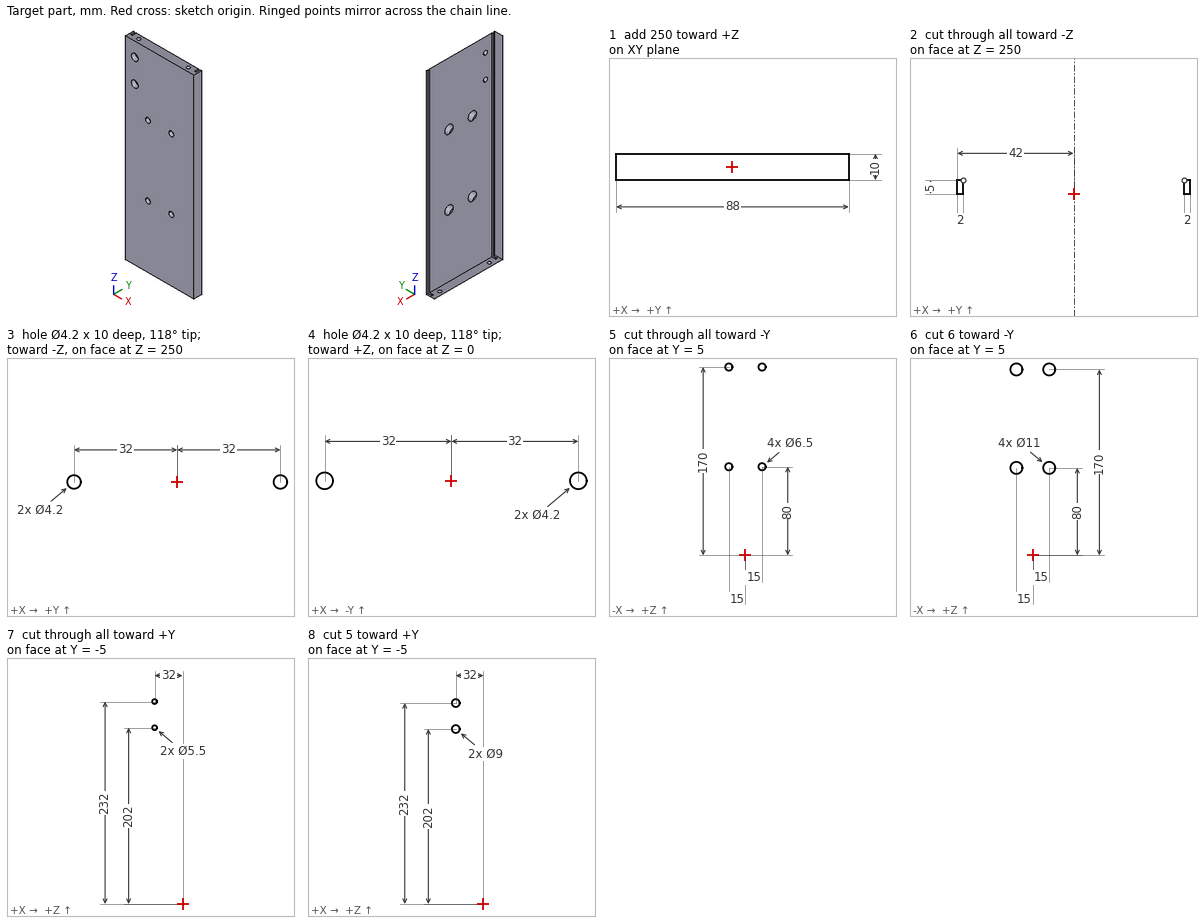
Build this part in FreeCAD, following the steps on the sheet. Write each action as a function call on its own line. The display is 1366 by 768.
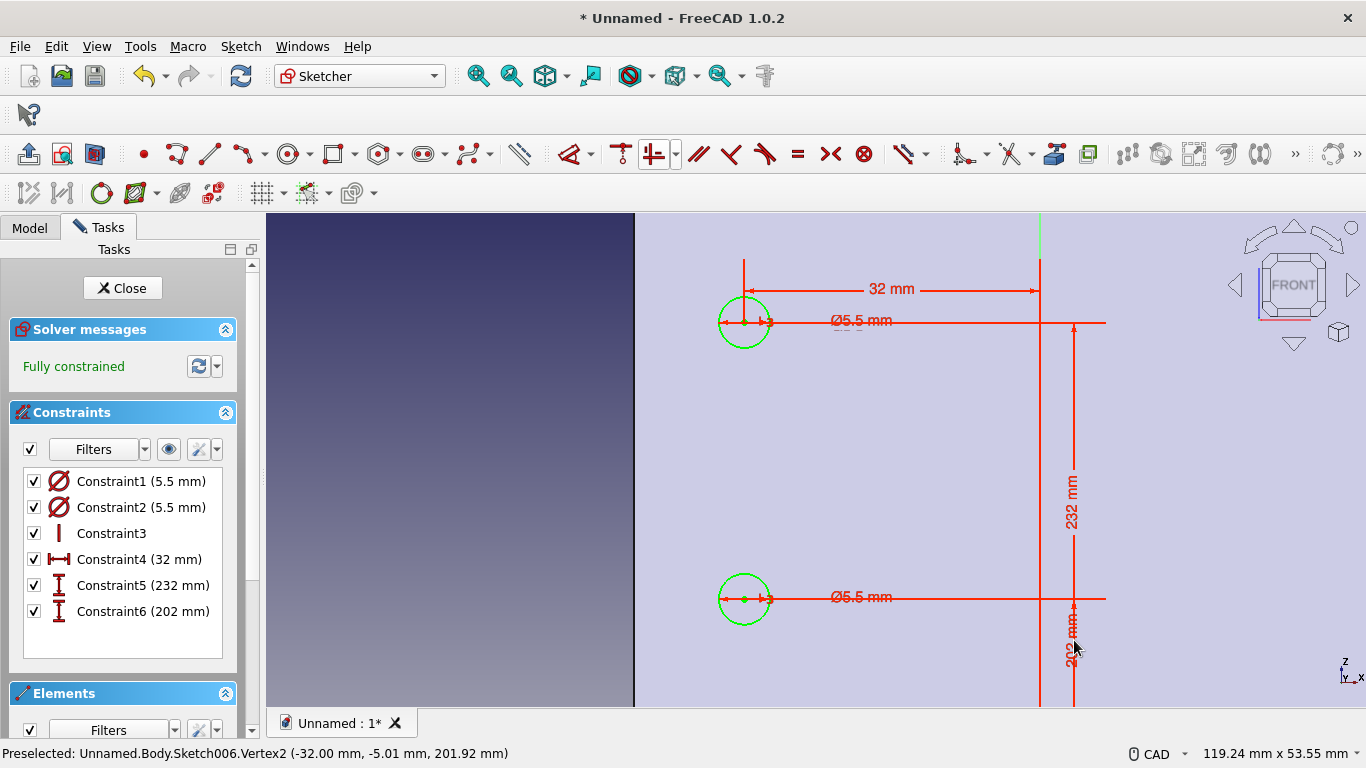
click(123, 288)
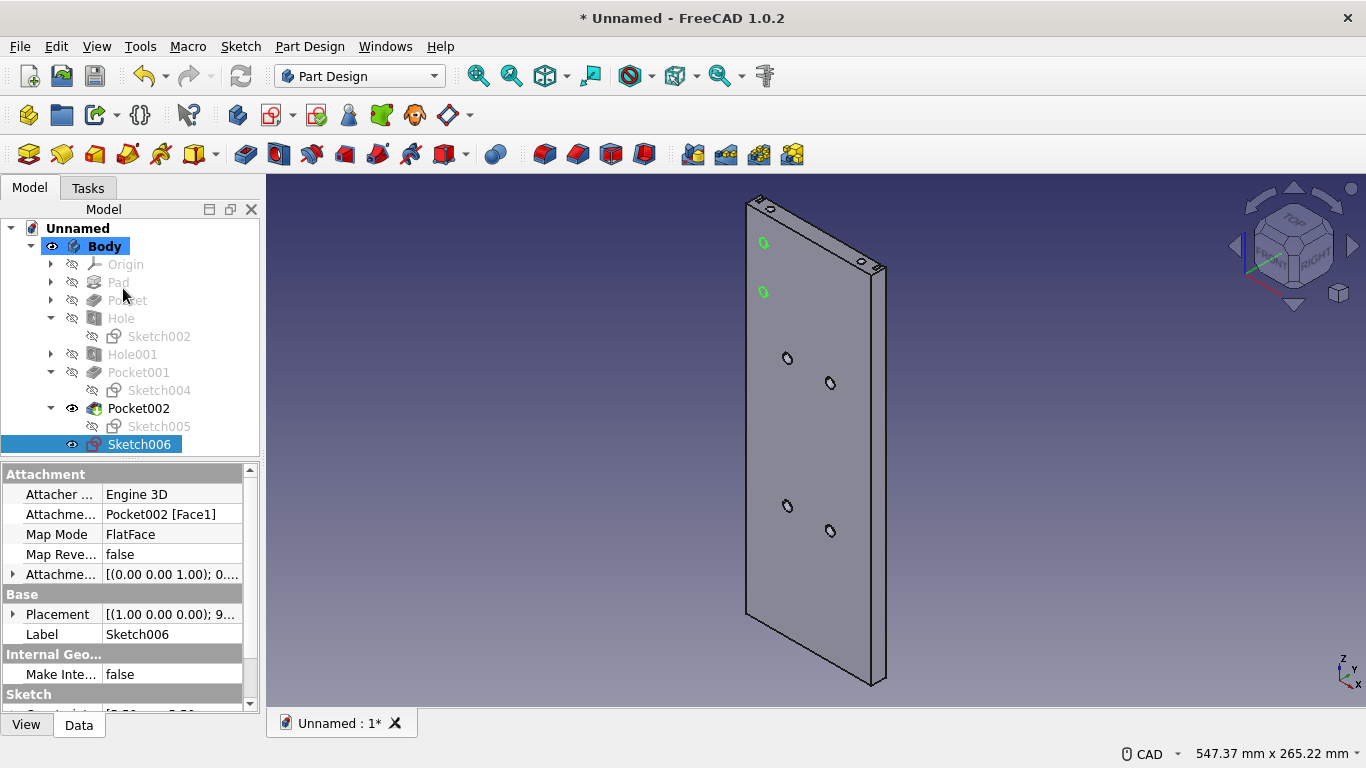
click(246, 154)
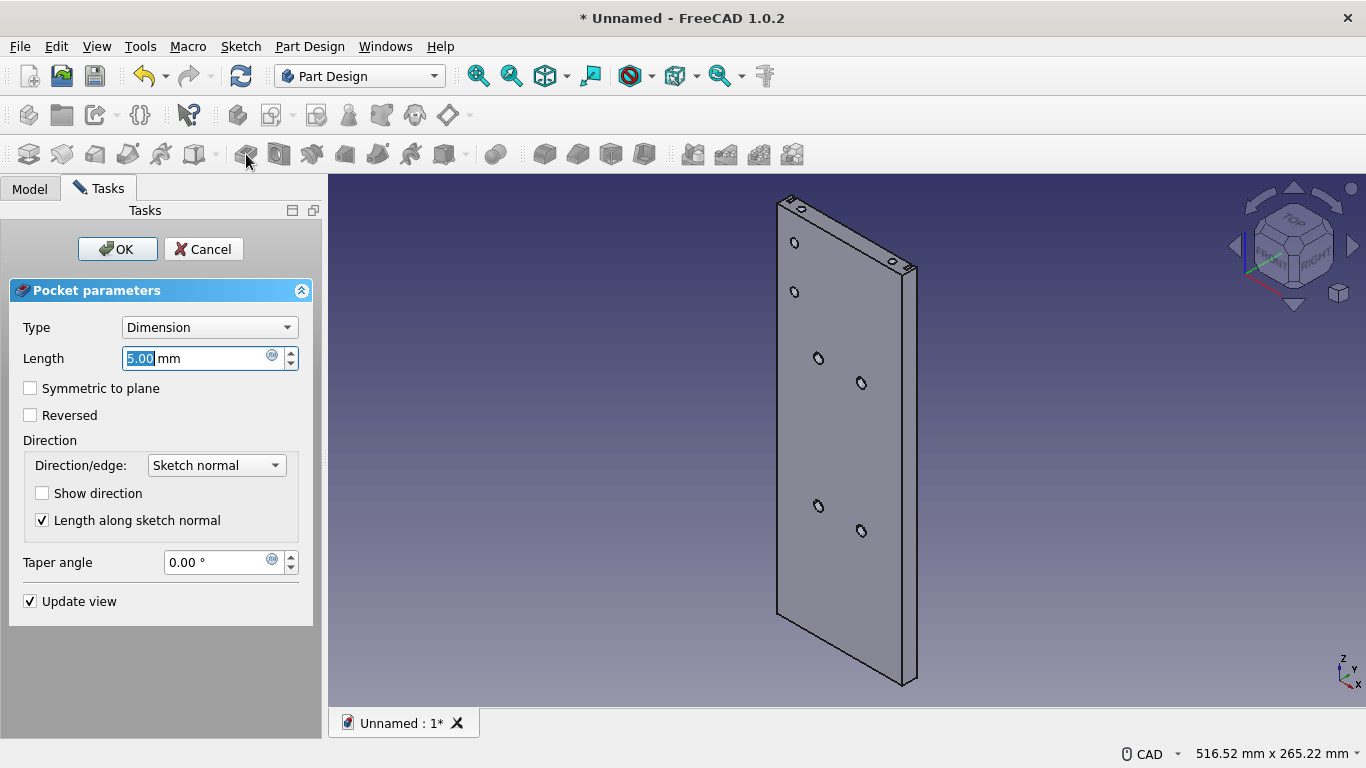
click(210, 328)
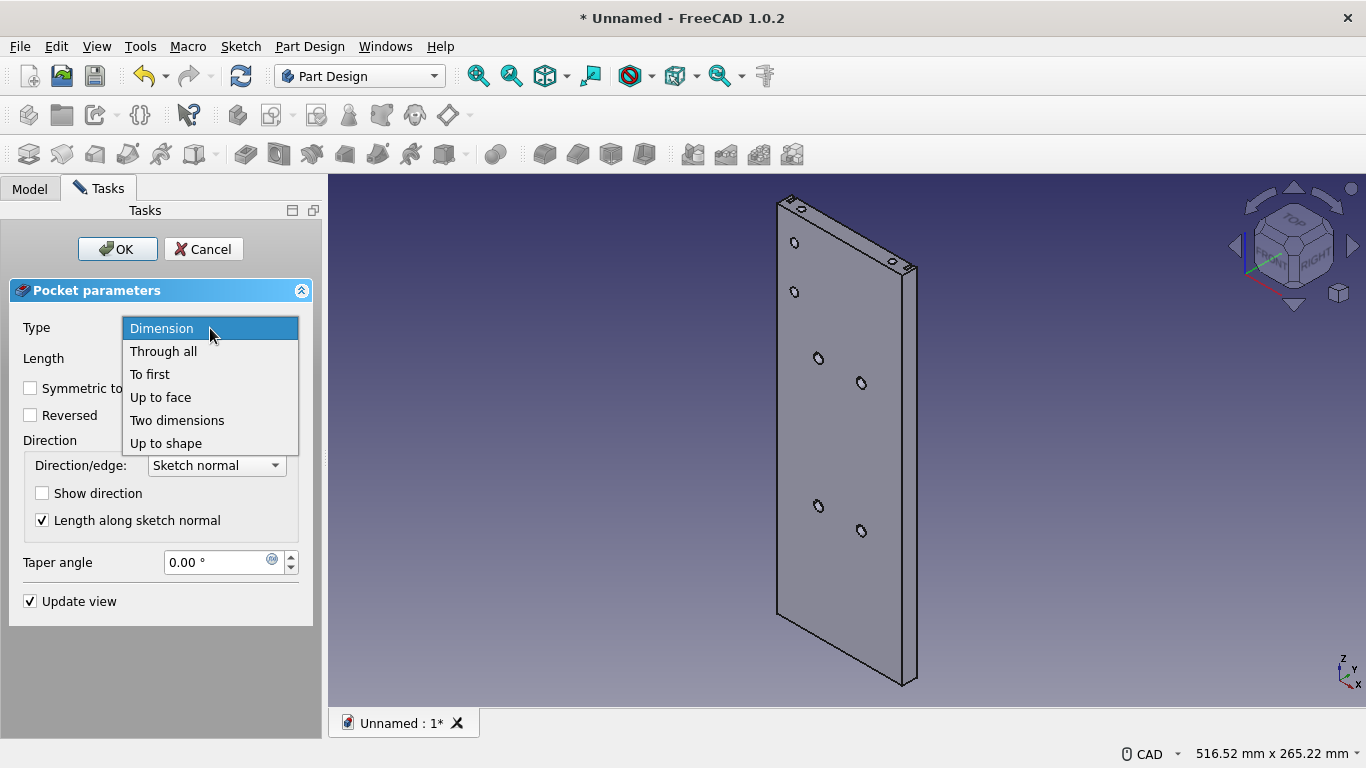
click(208, 352)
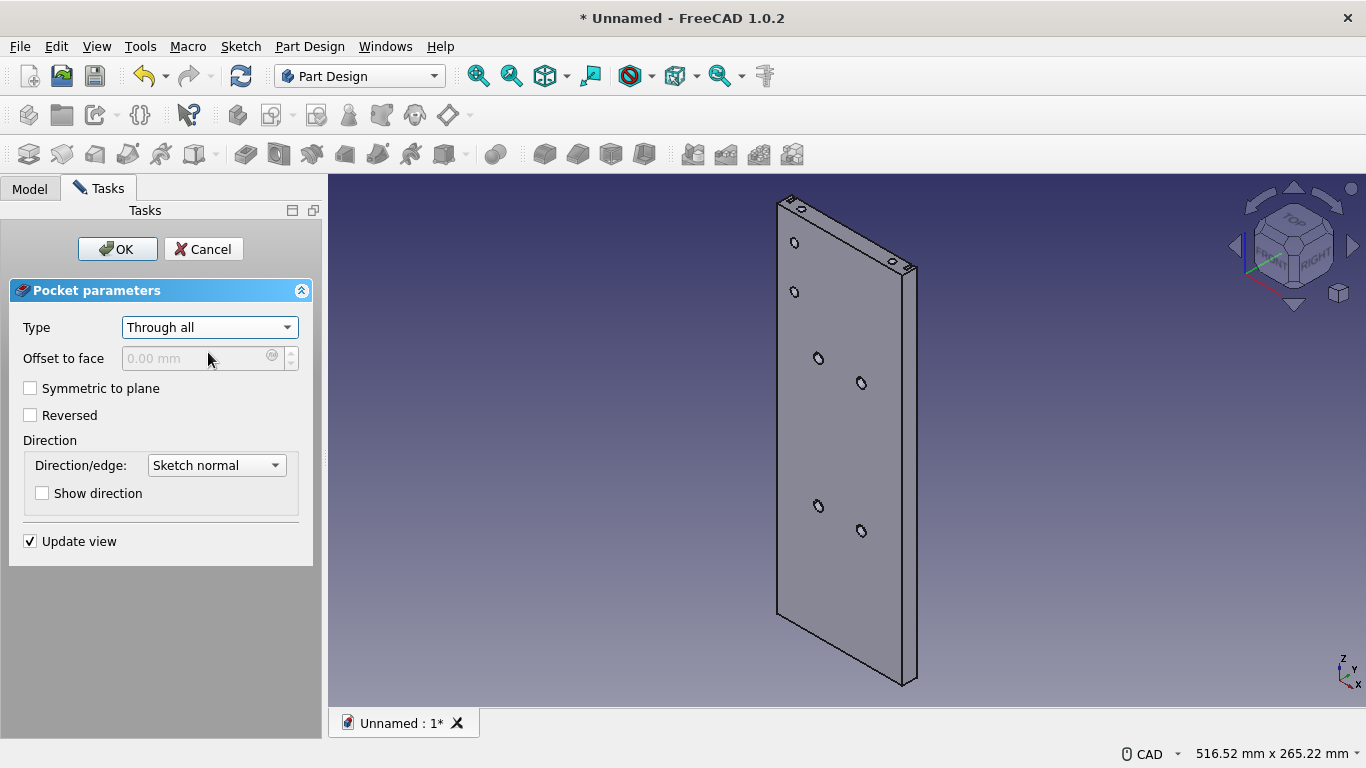
click(118, 249)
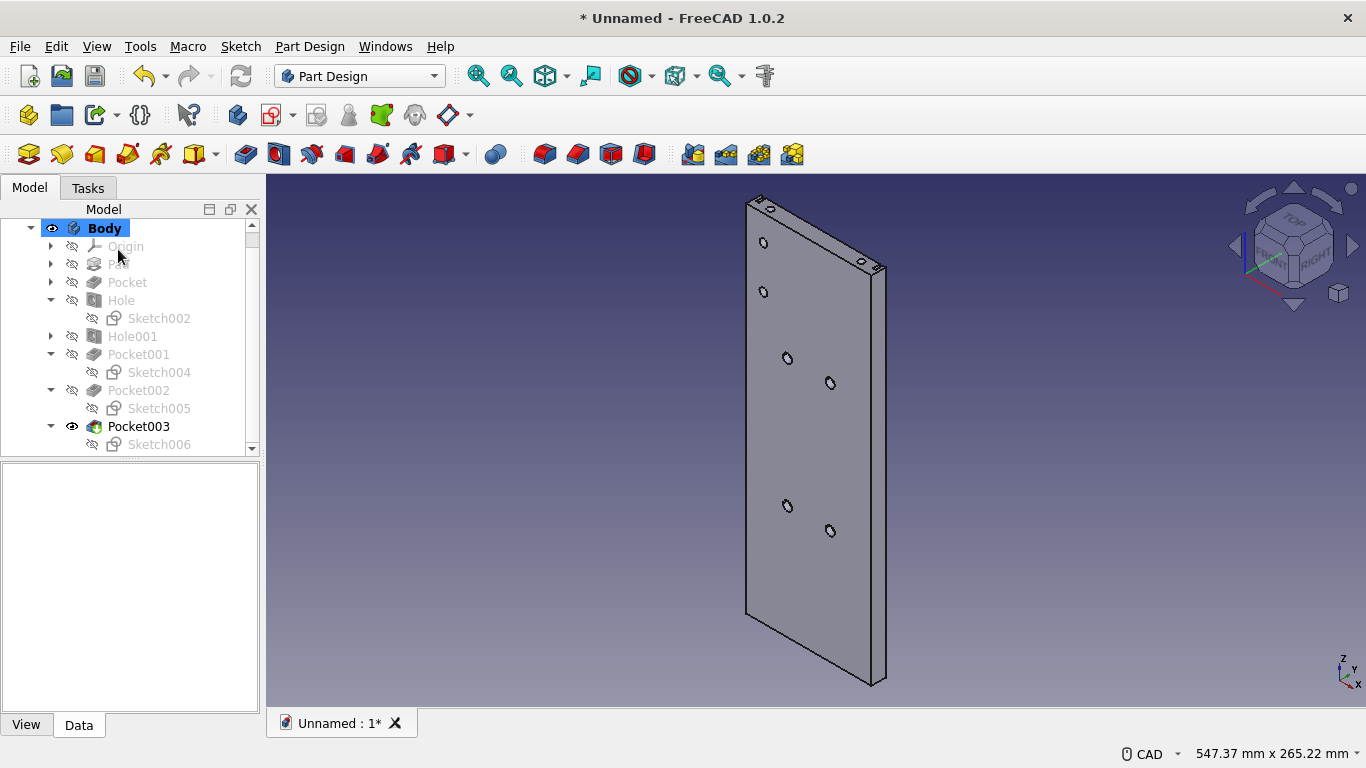
click(809, 444)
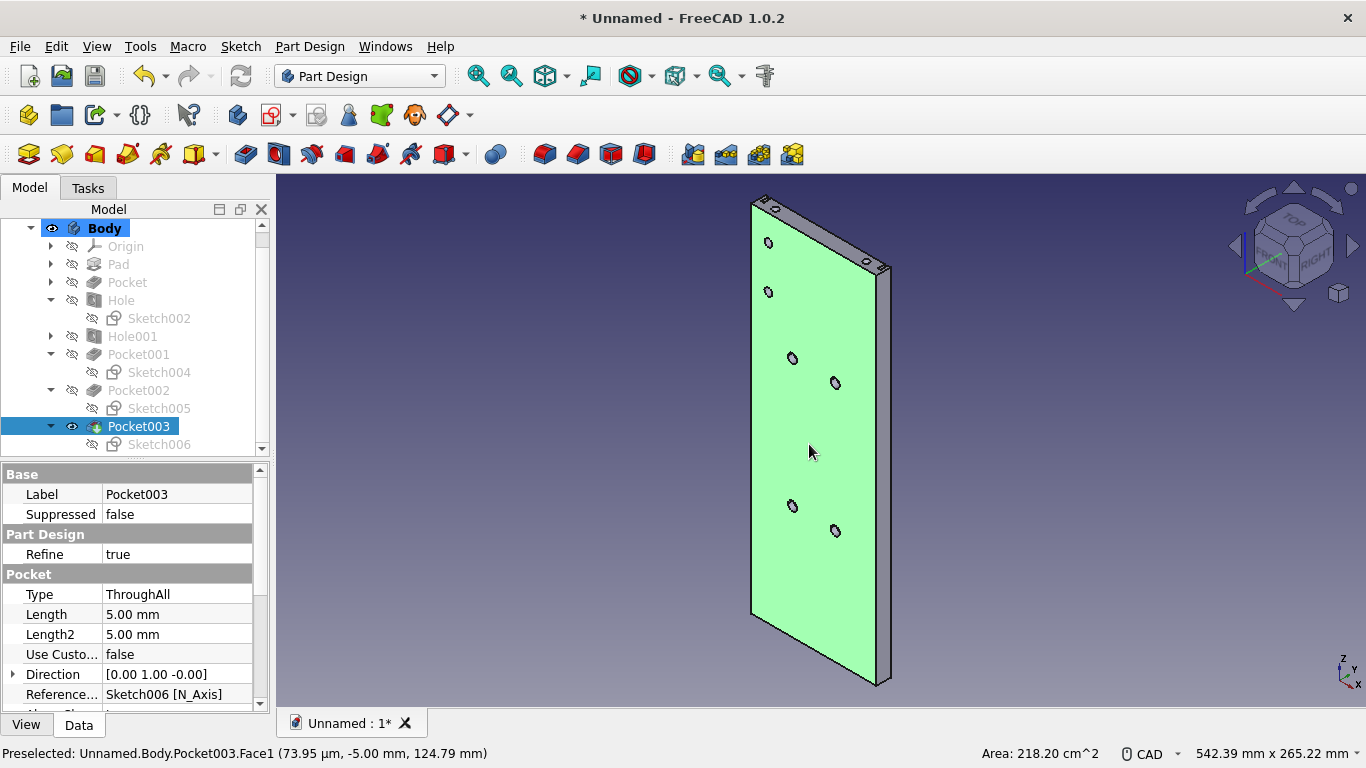
click(270, 116)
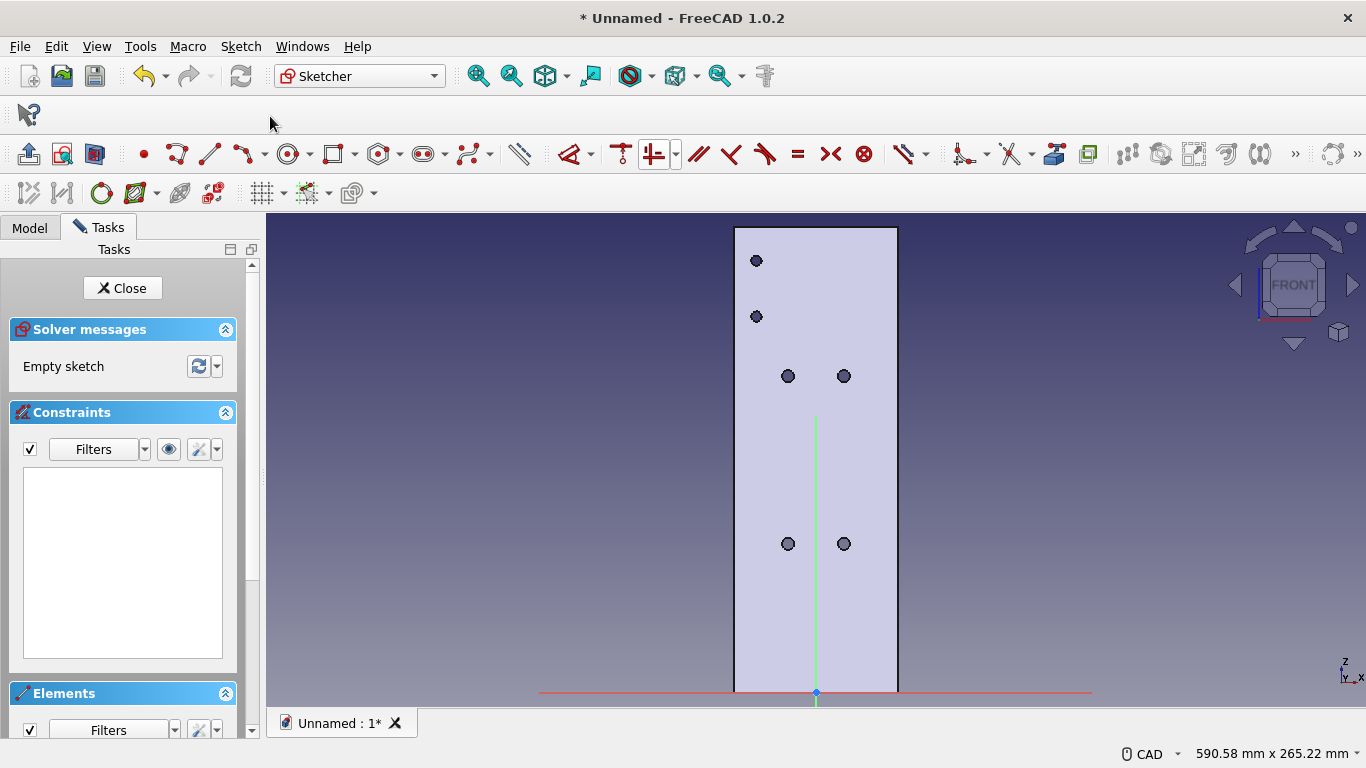
scroll(759, 241, up, 7)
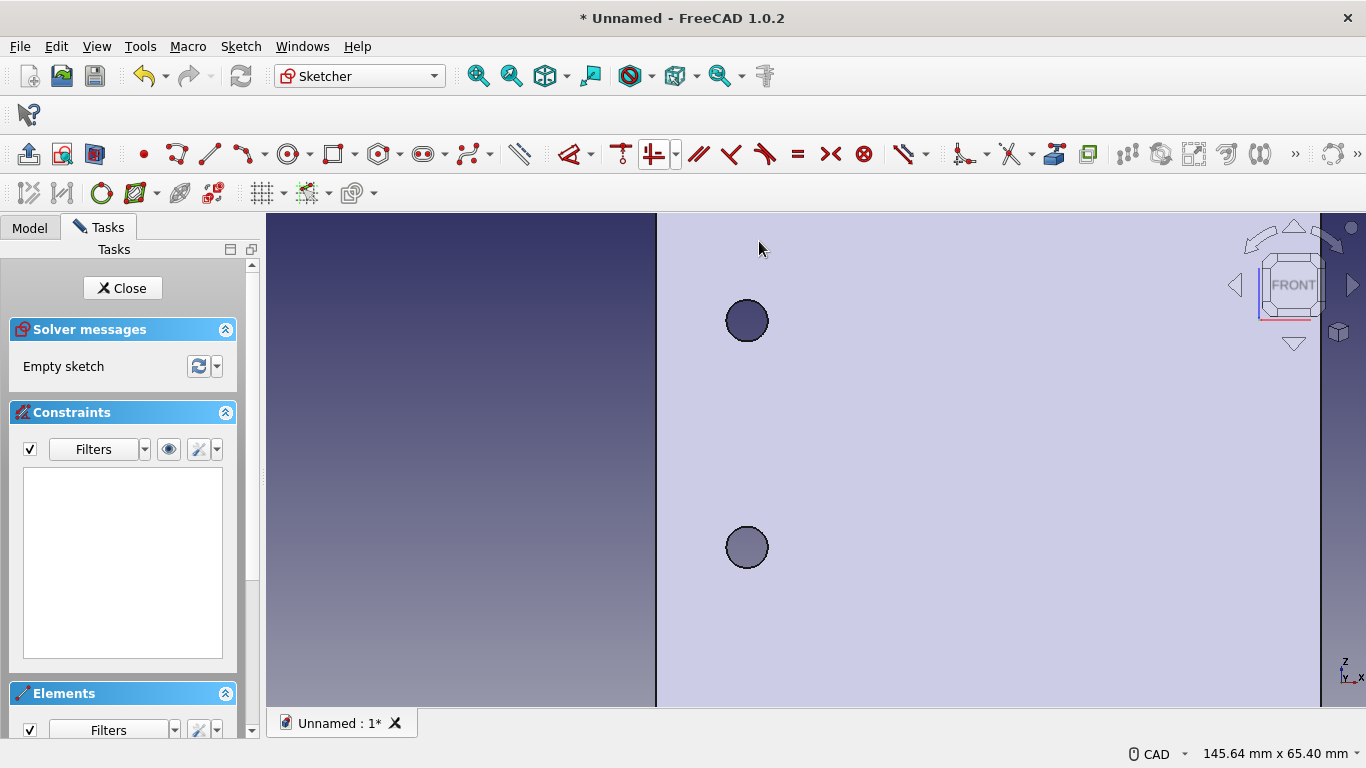
click(288, 154)